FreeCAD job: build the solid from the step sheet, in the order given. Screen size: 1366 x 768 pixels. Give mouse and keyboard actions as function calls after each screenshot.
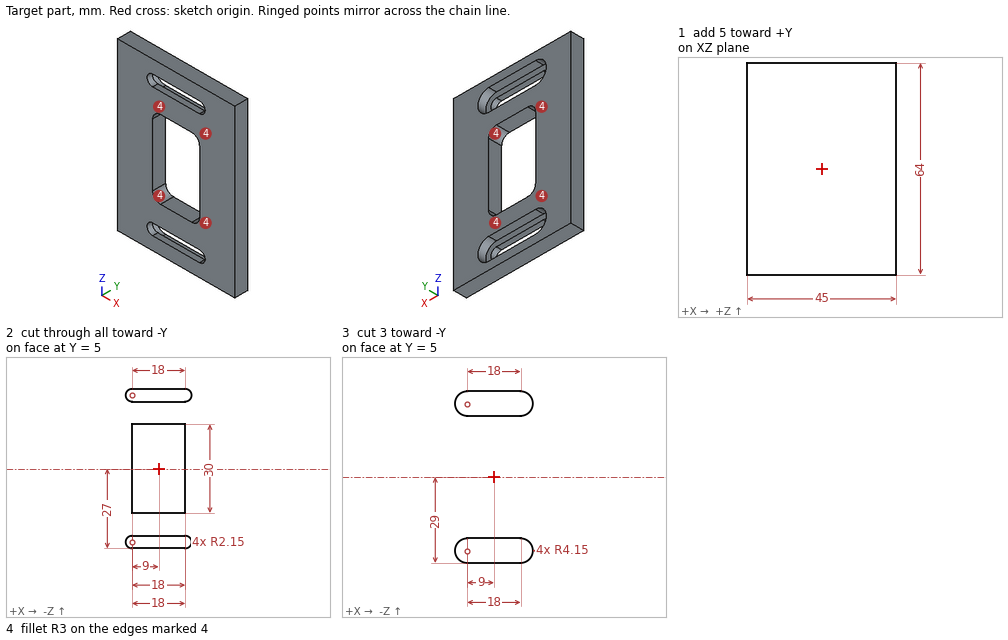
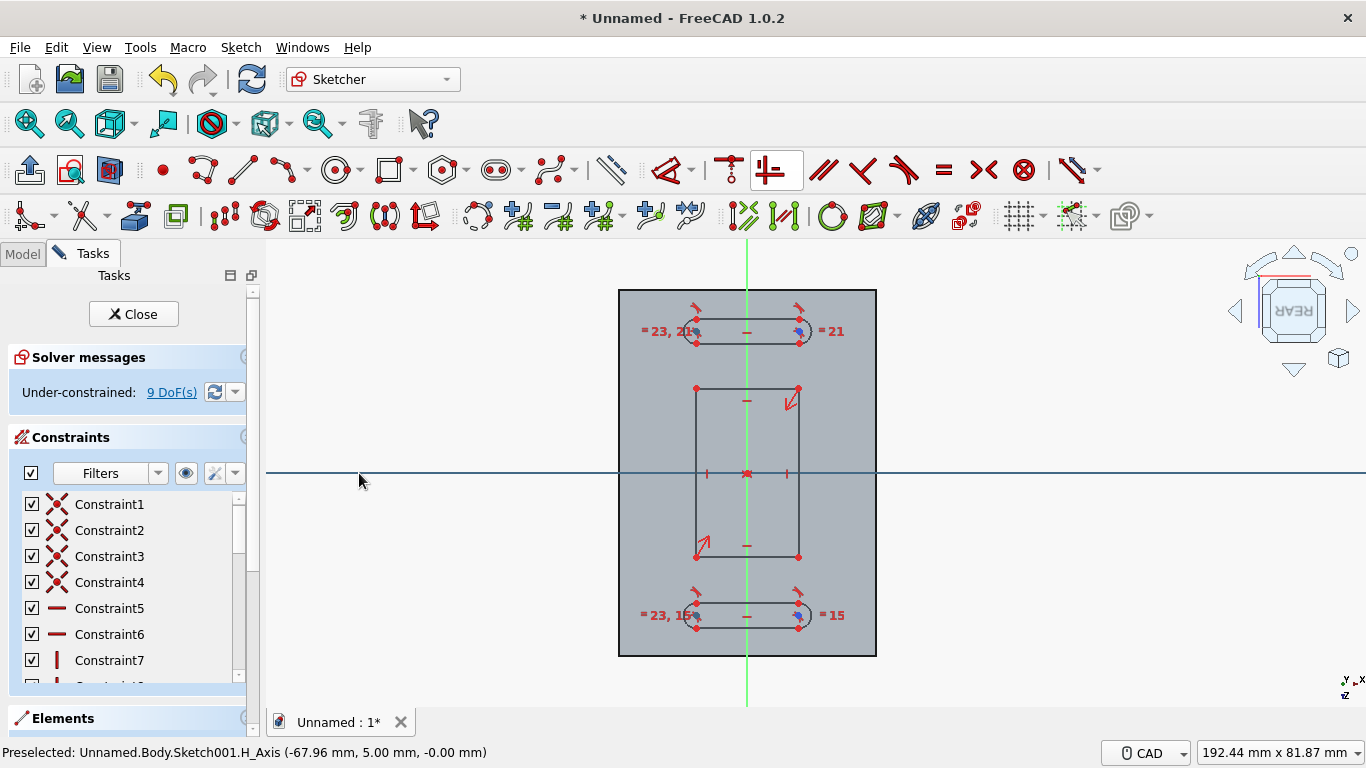
click(984, 170)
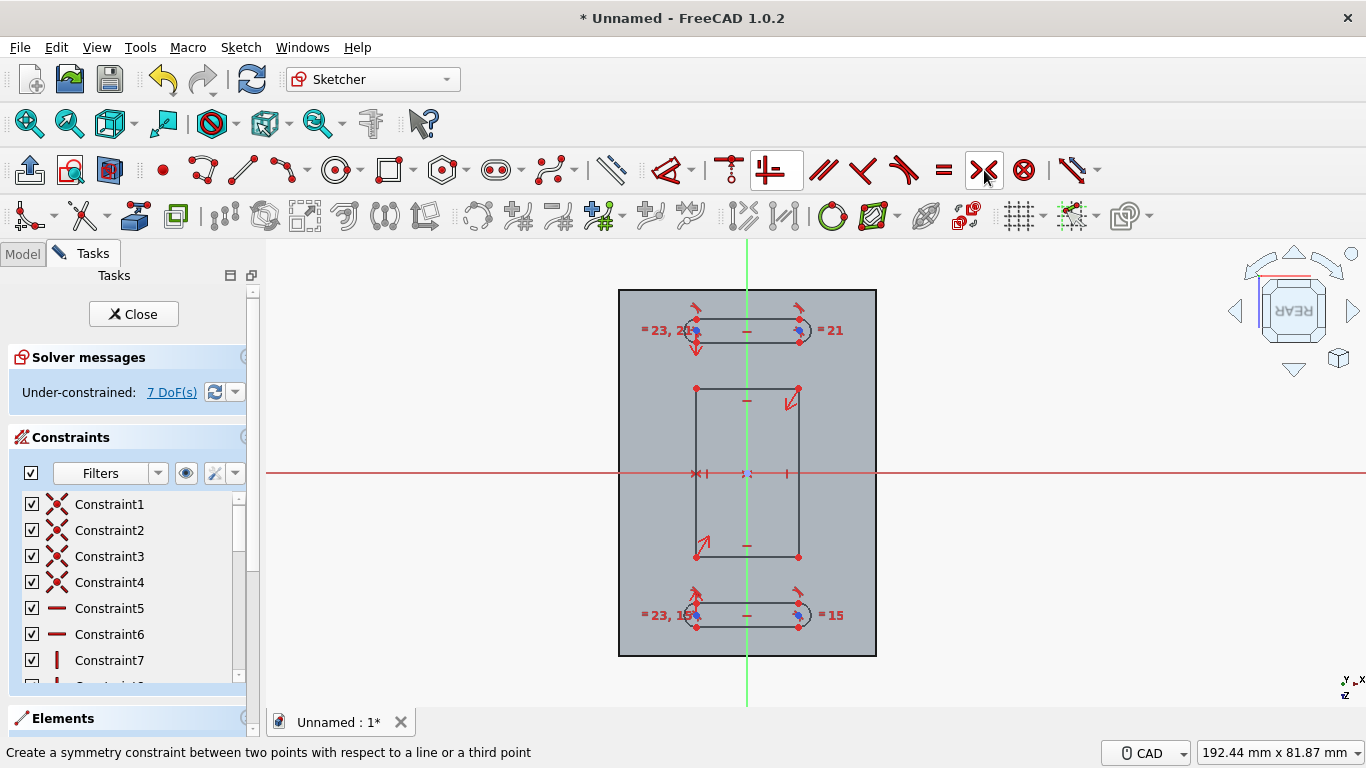
click(666, 170)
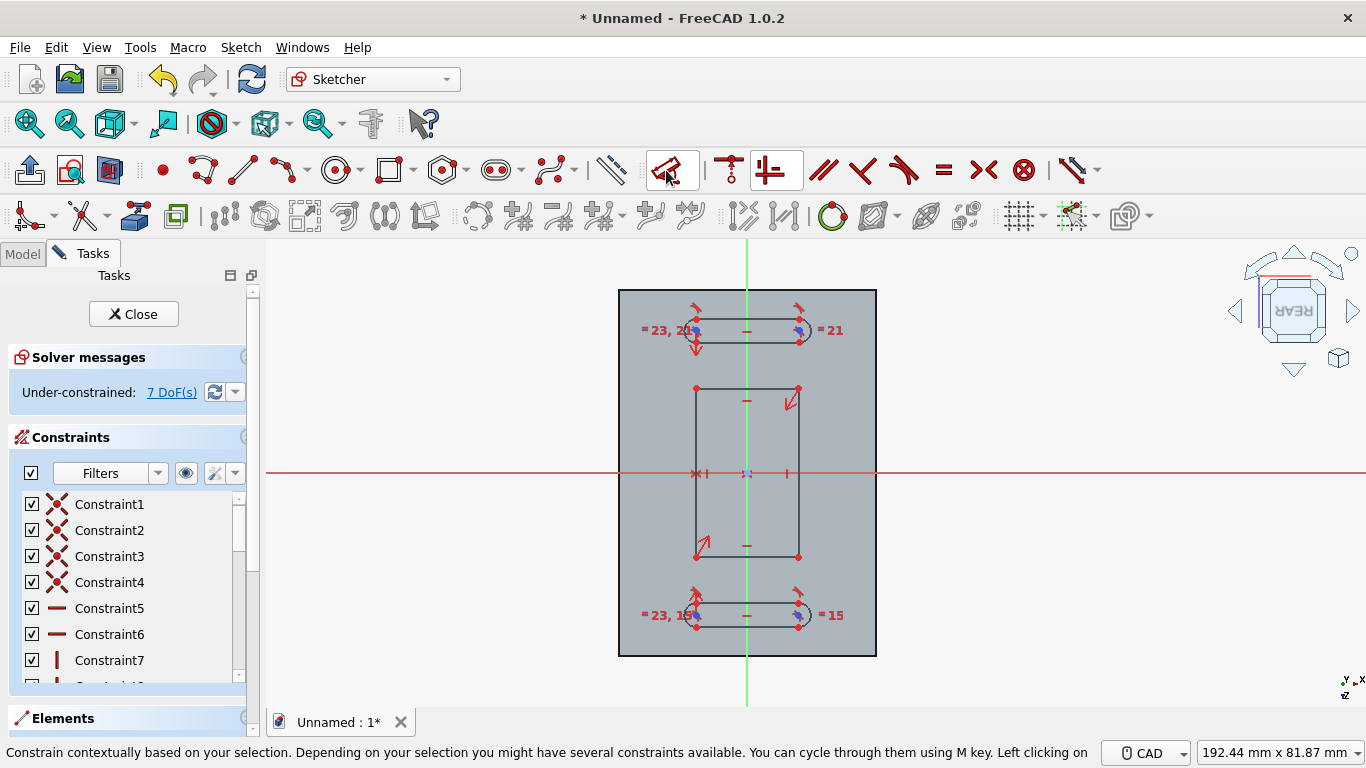
scroll(687, 608, up, 6)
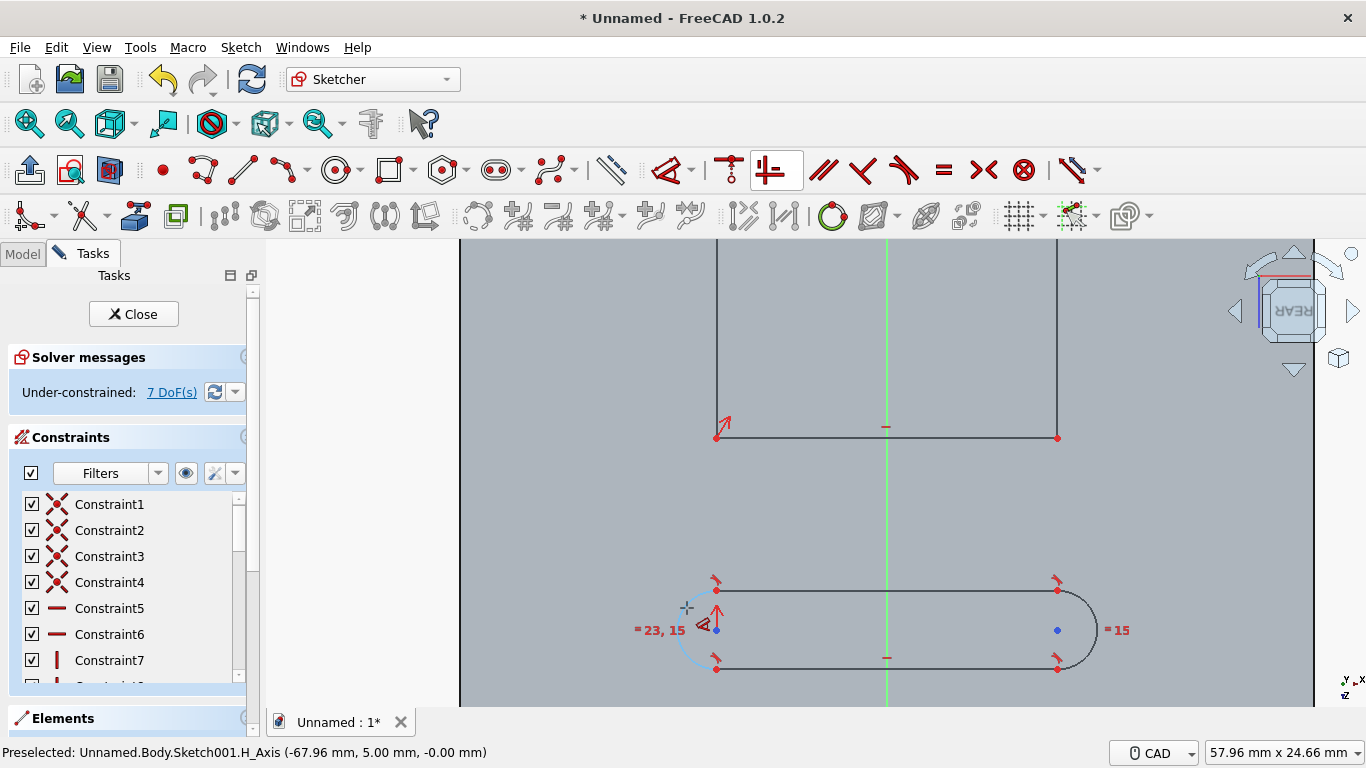
click(685, 607)
click(659, 588)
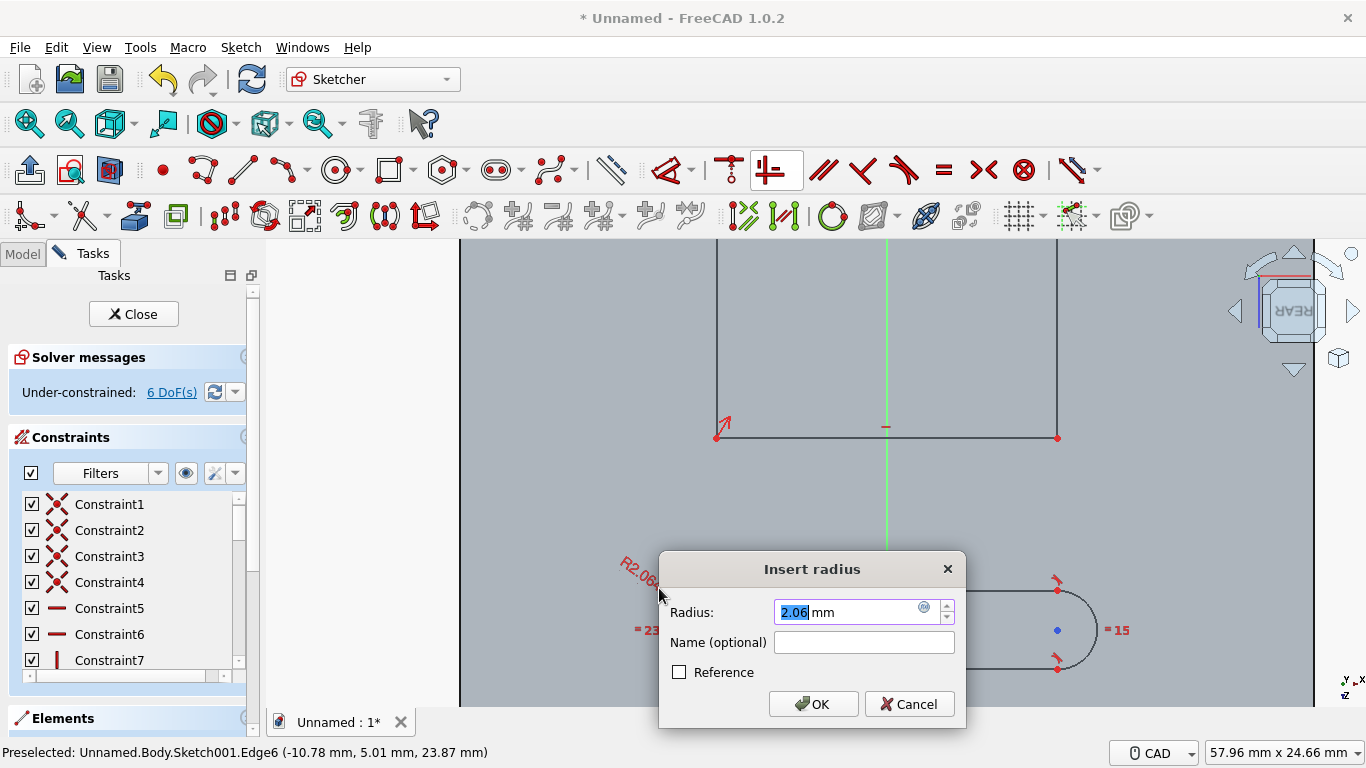
text(2.15)
key(Return)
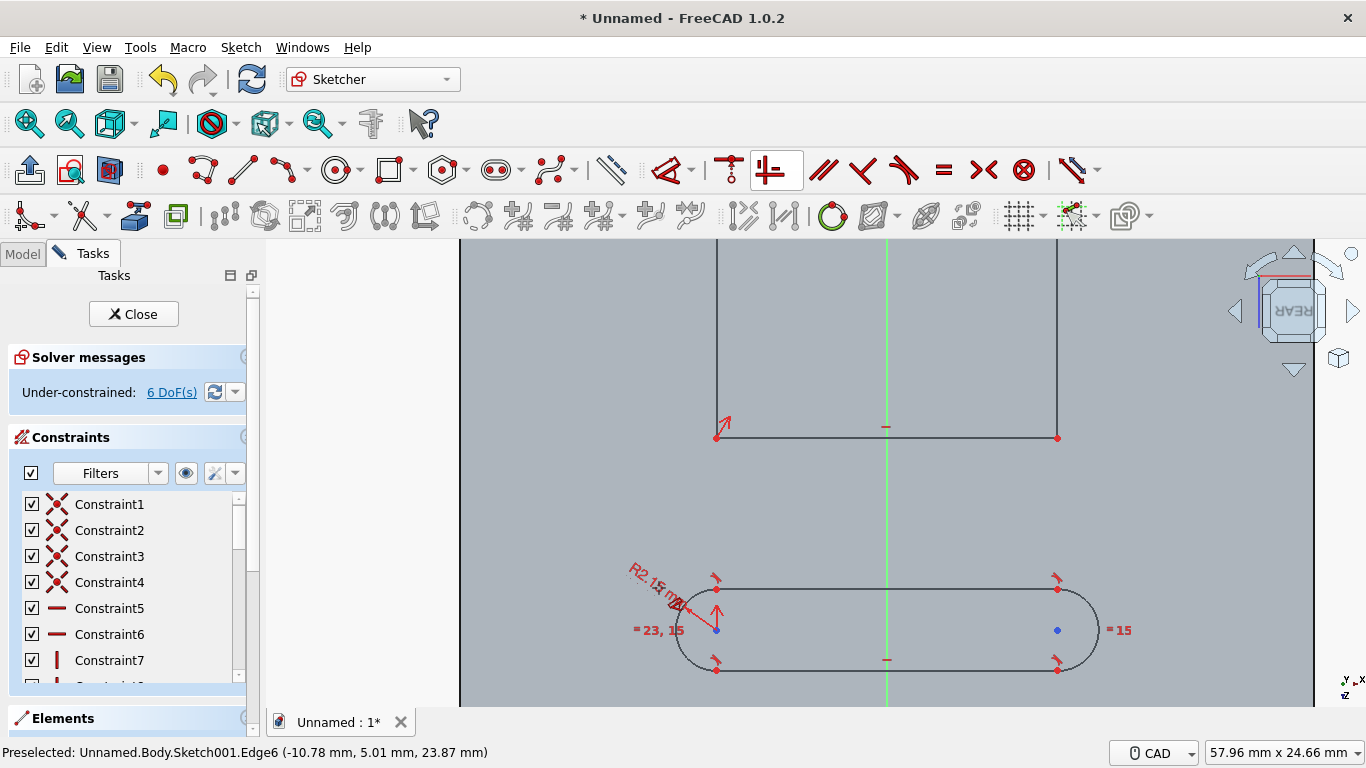
scroll(687, 609, down, 6)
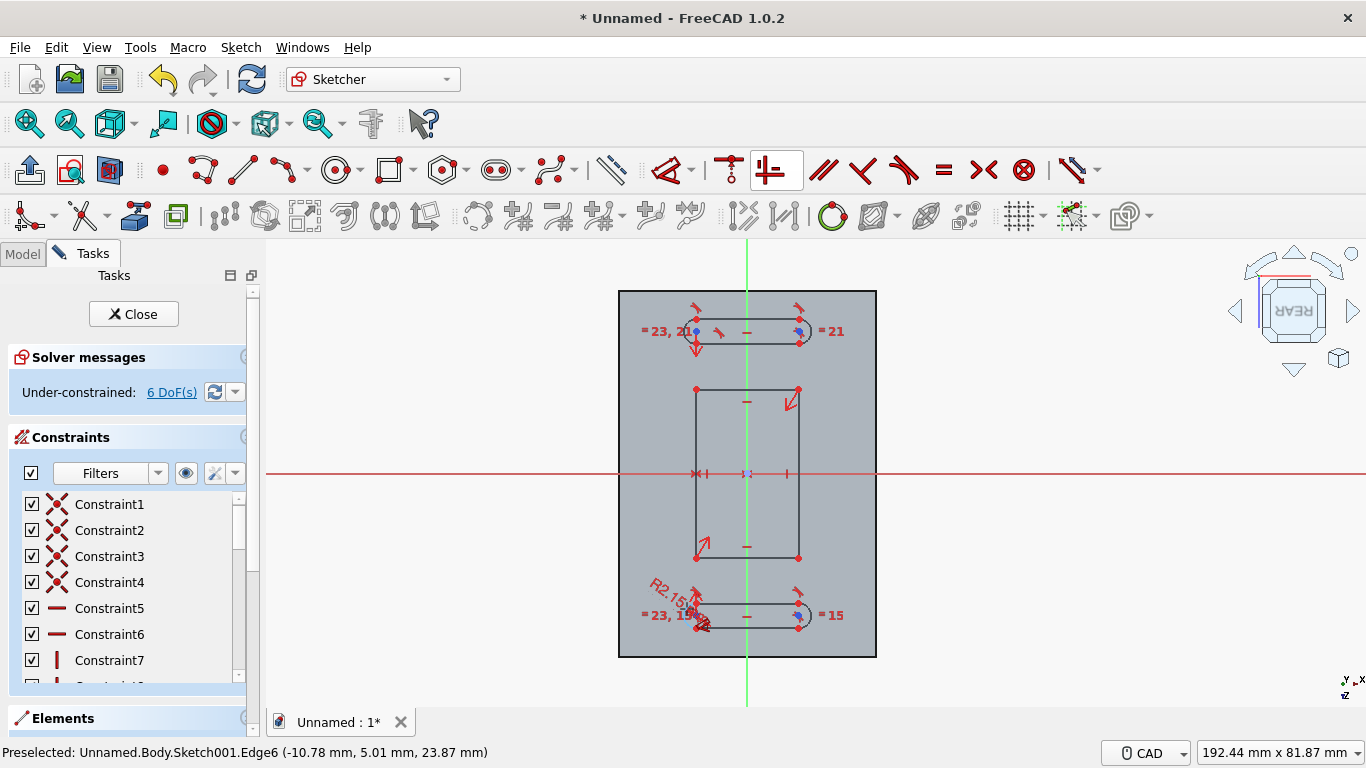
click(727, 558)
click(724, 524)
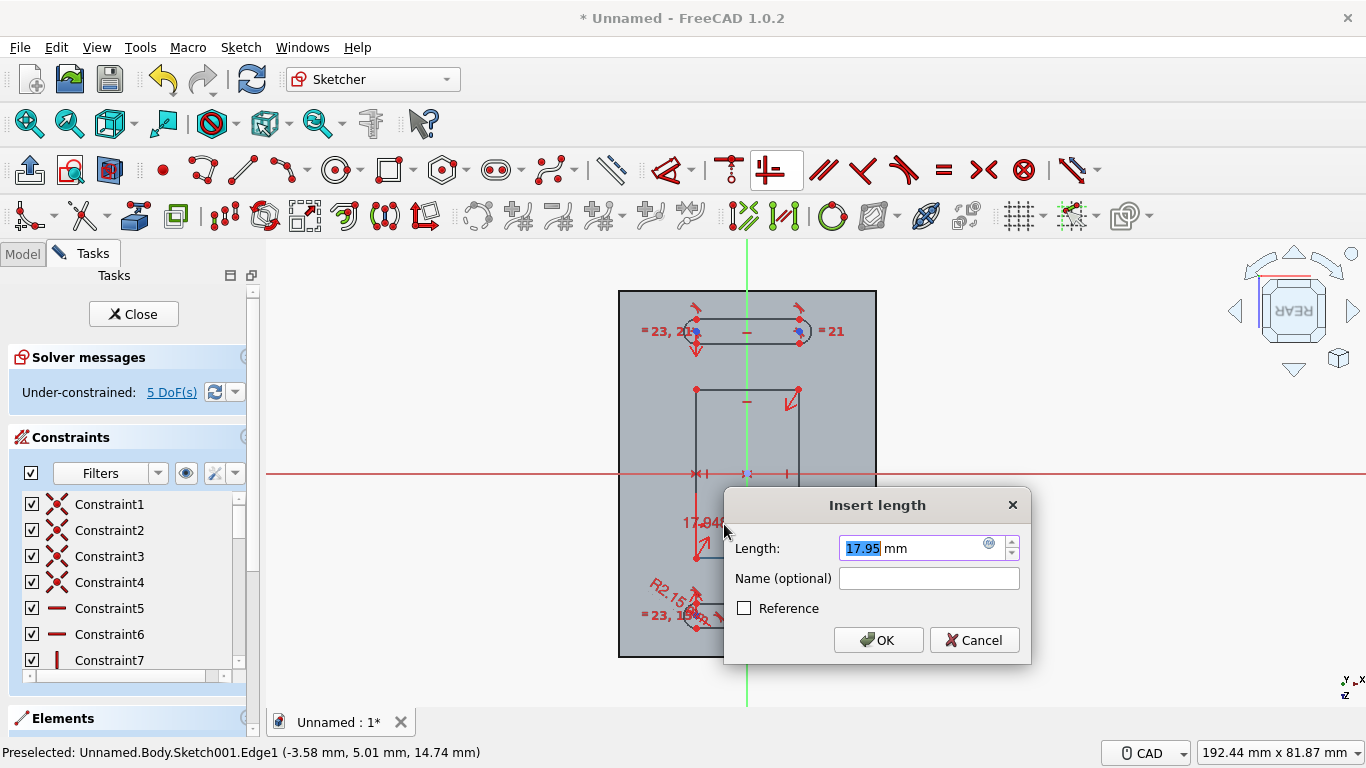
text(18)
key(Return)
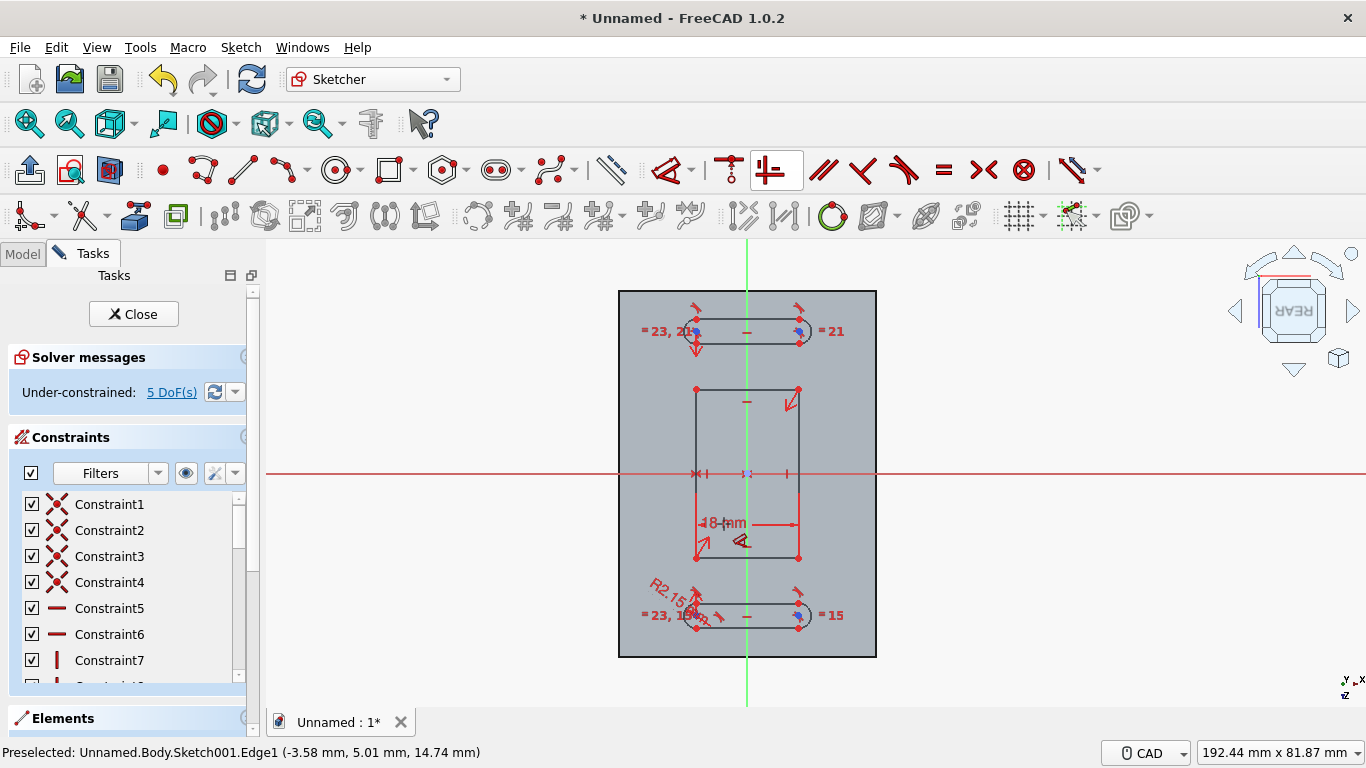
click(799, 507)
click(833, 435)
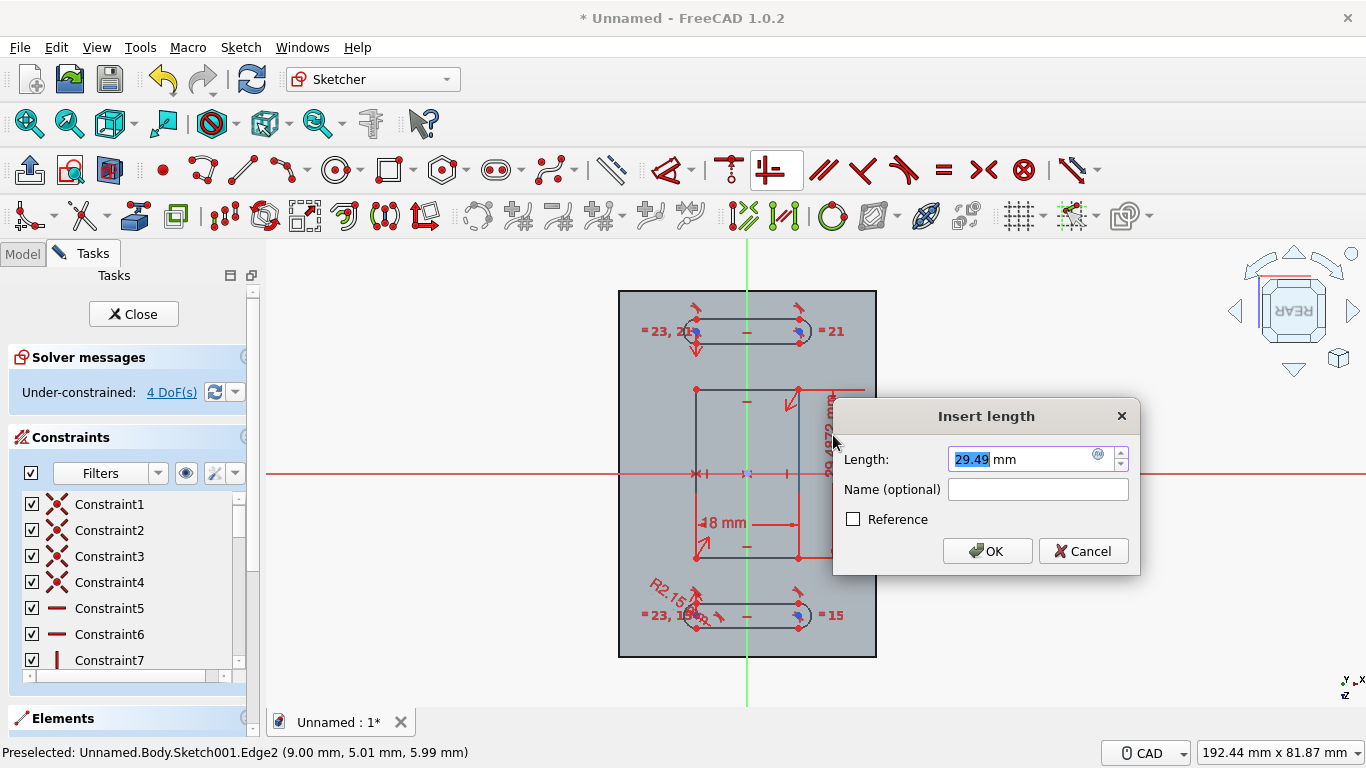
text(30)
key(Return)